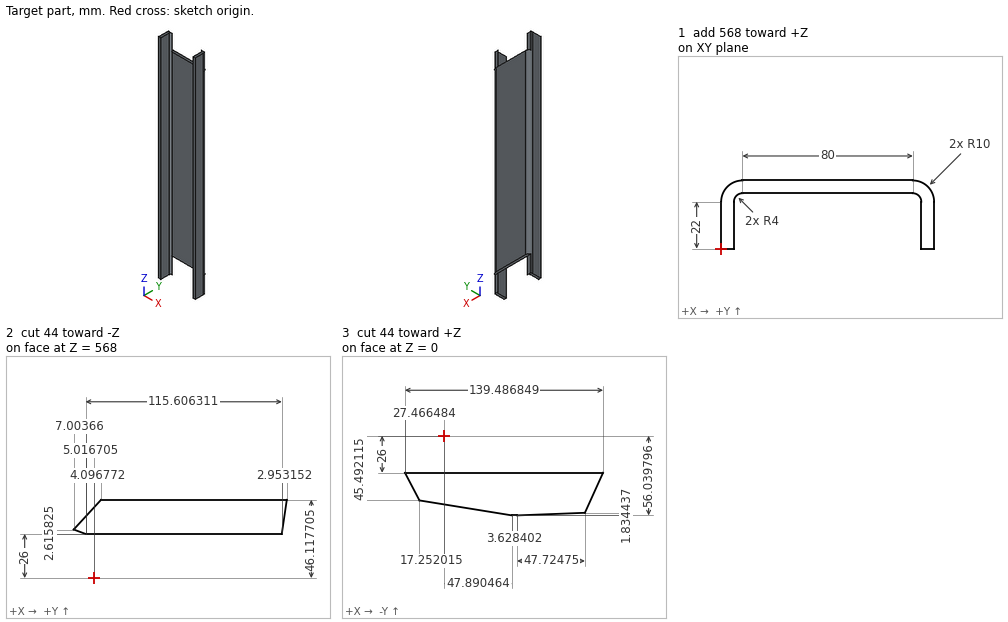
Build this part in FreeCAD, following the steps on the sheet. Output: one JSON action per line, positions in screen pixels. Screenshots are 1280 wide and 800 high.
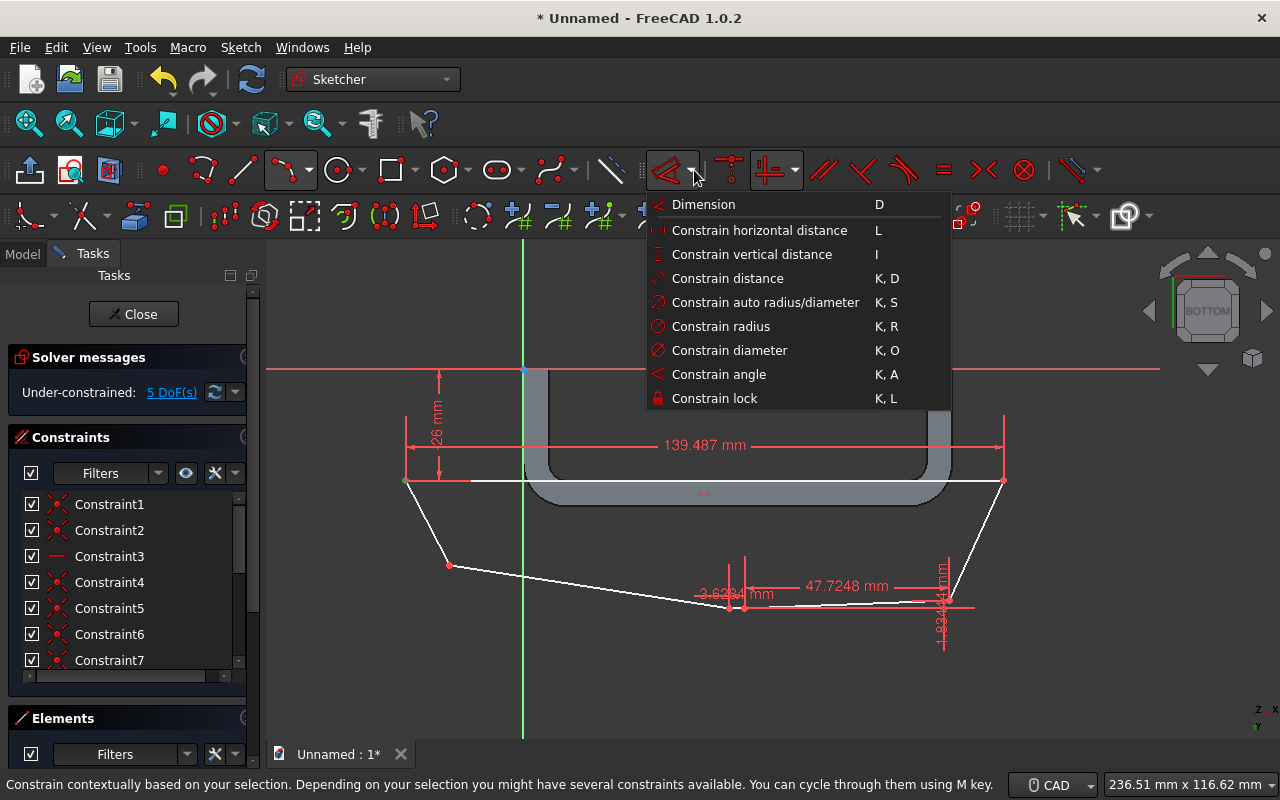
{"action": "left_click", "coordinate": [799, 230]}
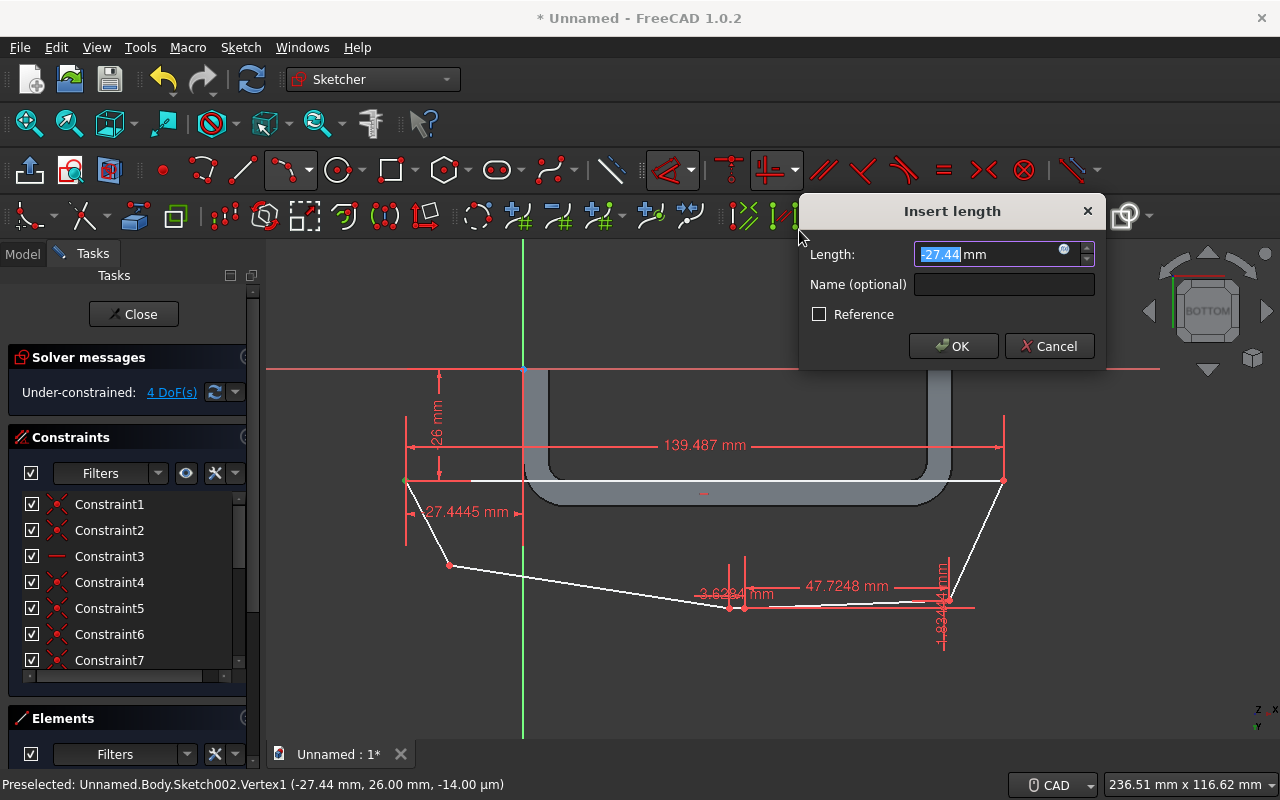
{"action": "type", "text": "-27.466484"}
{"action": "key", "text": "Return"}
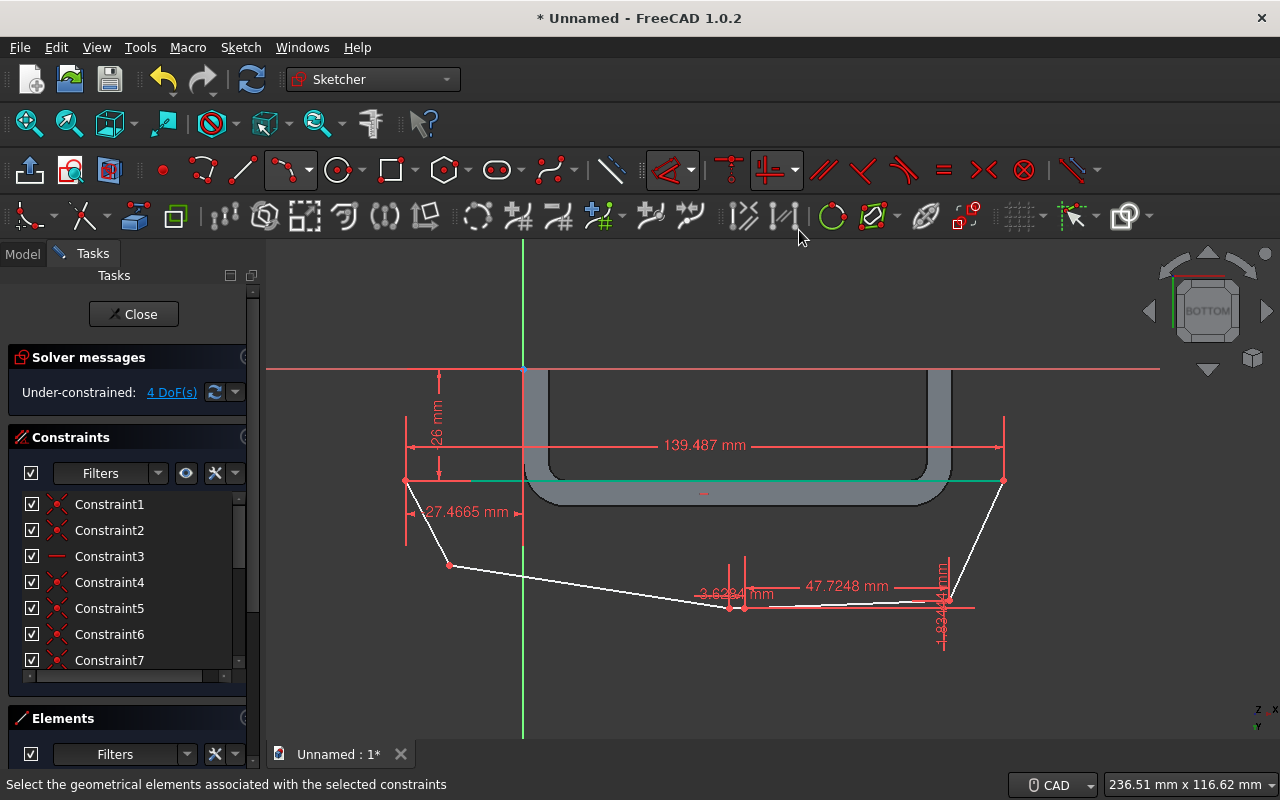
{"action": "left_click", "coordinate": [450, 565]}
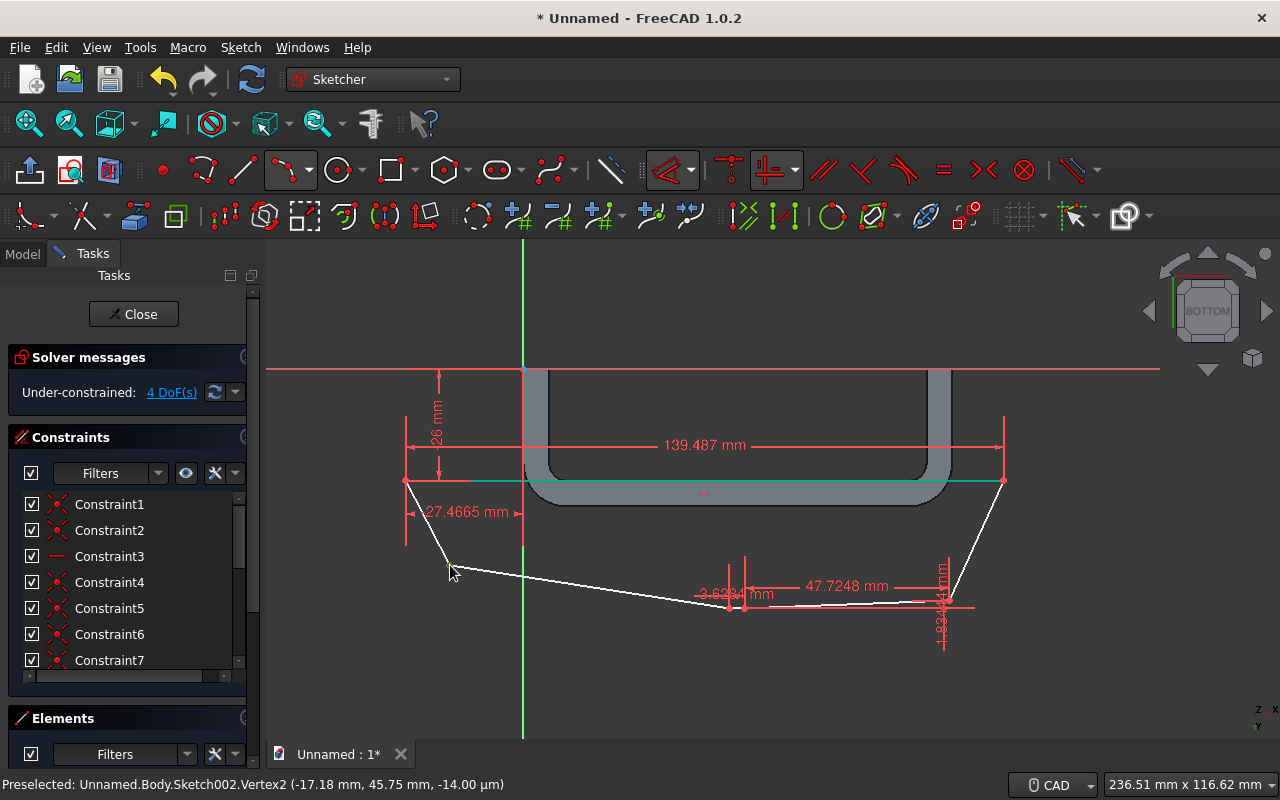
{"action": "key", "text": "l"}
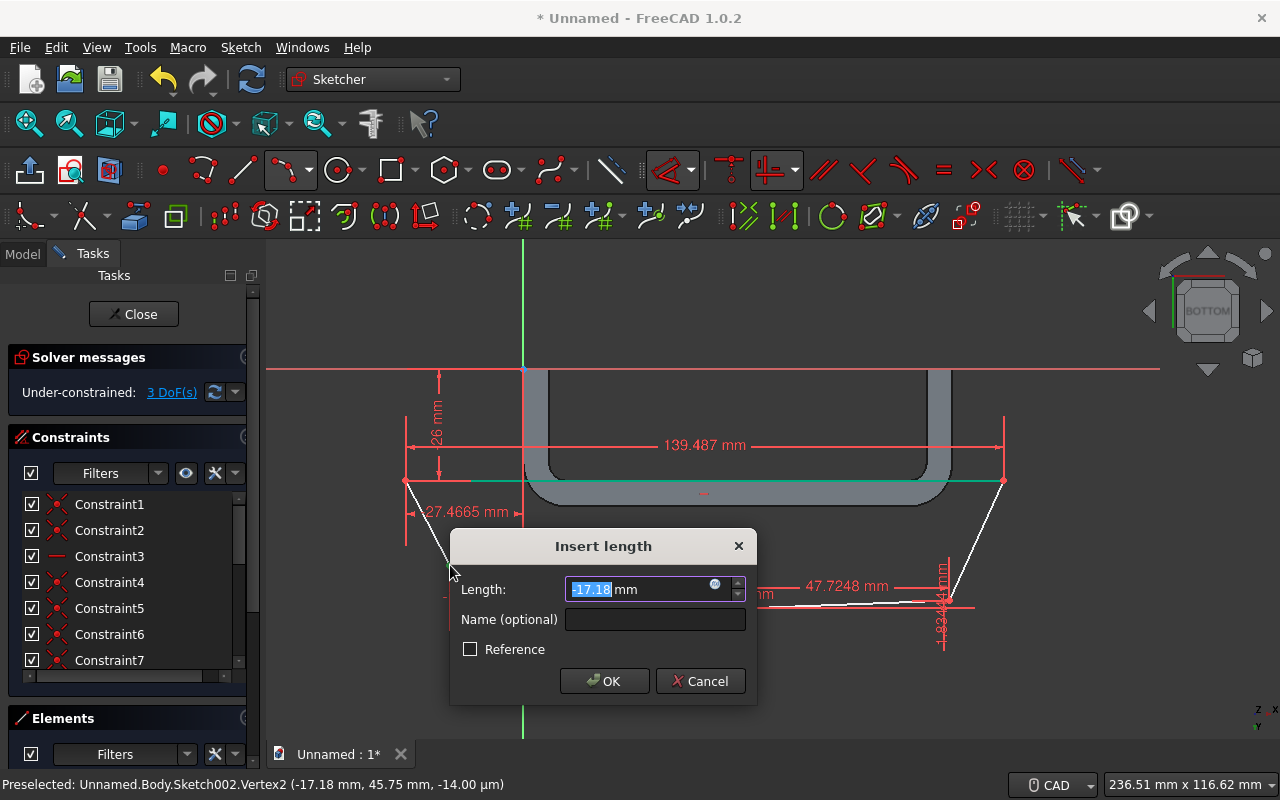
{"action": "type", "text": "-17.252015"}
{"action": "key", "text": "Return"}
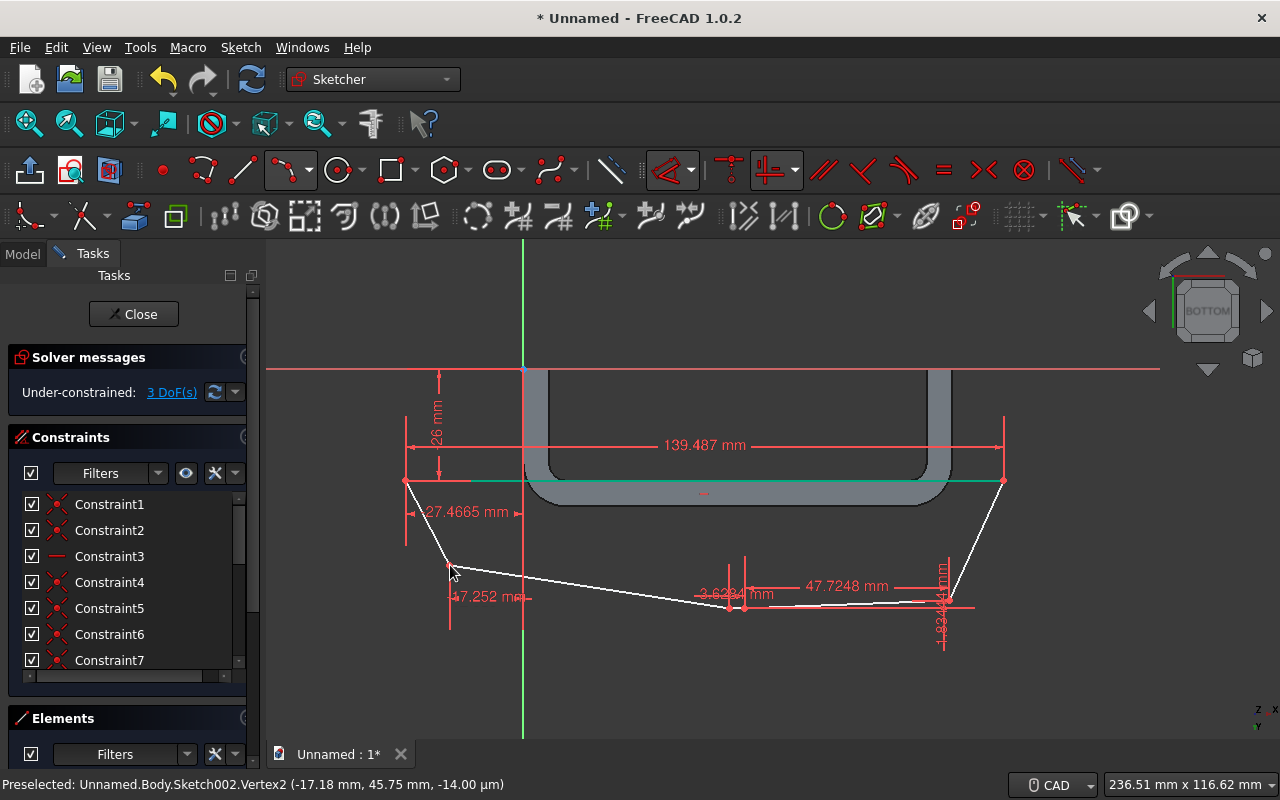
{"action": "left_click", "coordinate": [450, 565]}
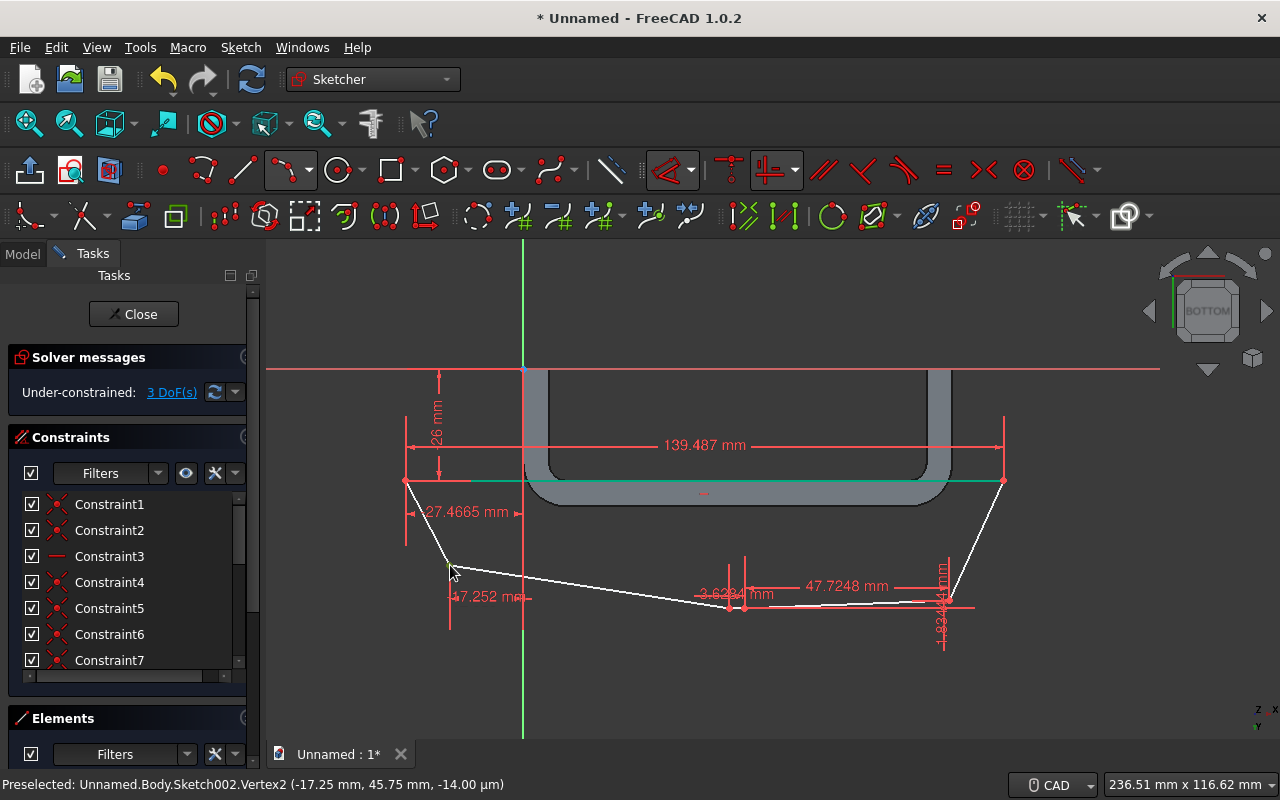
{"action": "key", "text": "i"}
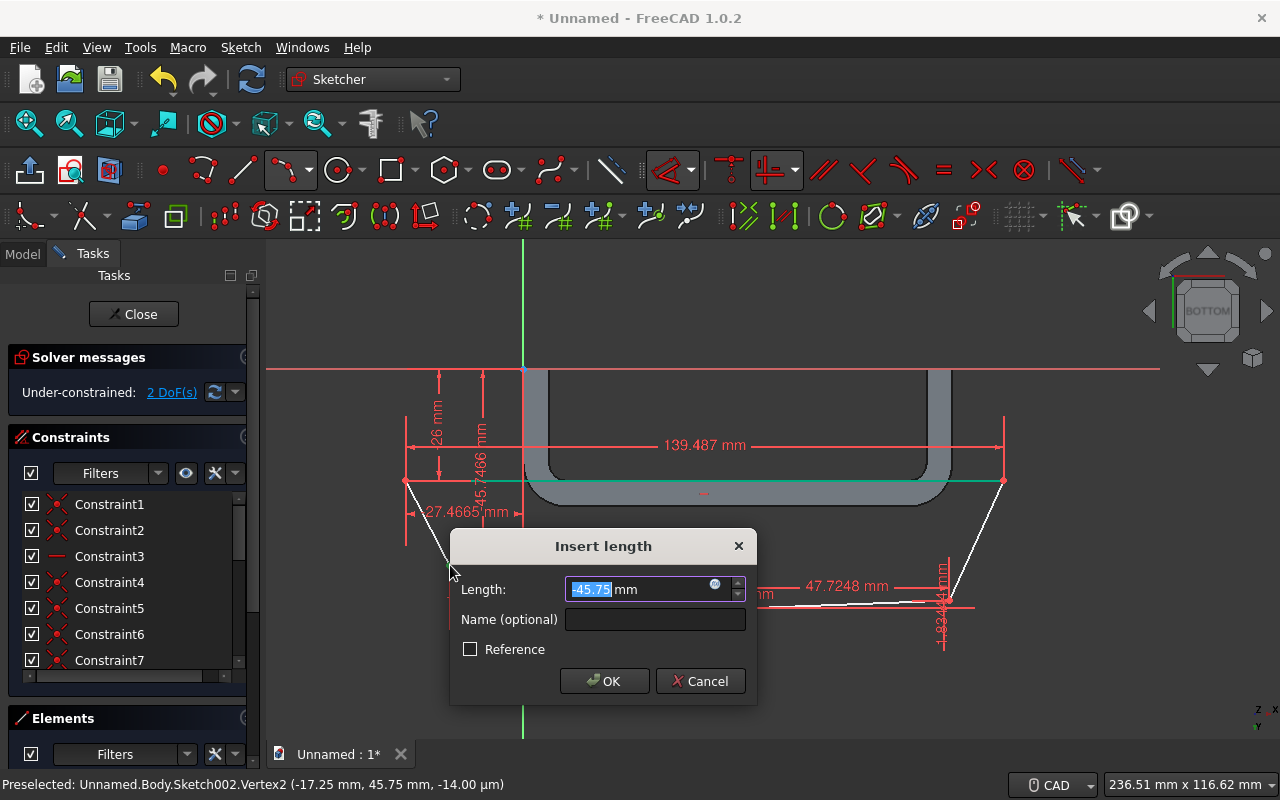
{"action": "type", "text": "-45.492115"}
{"action": "key", "text": "Return"}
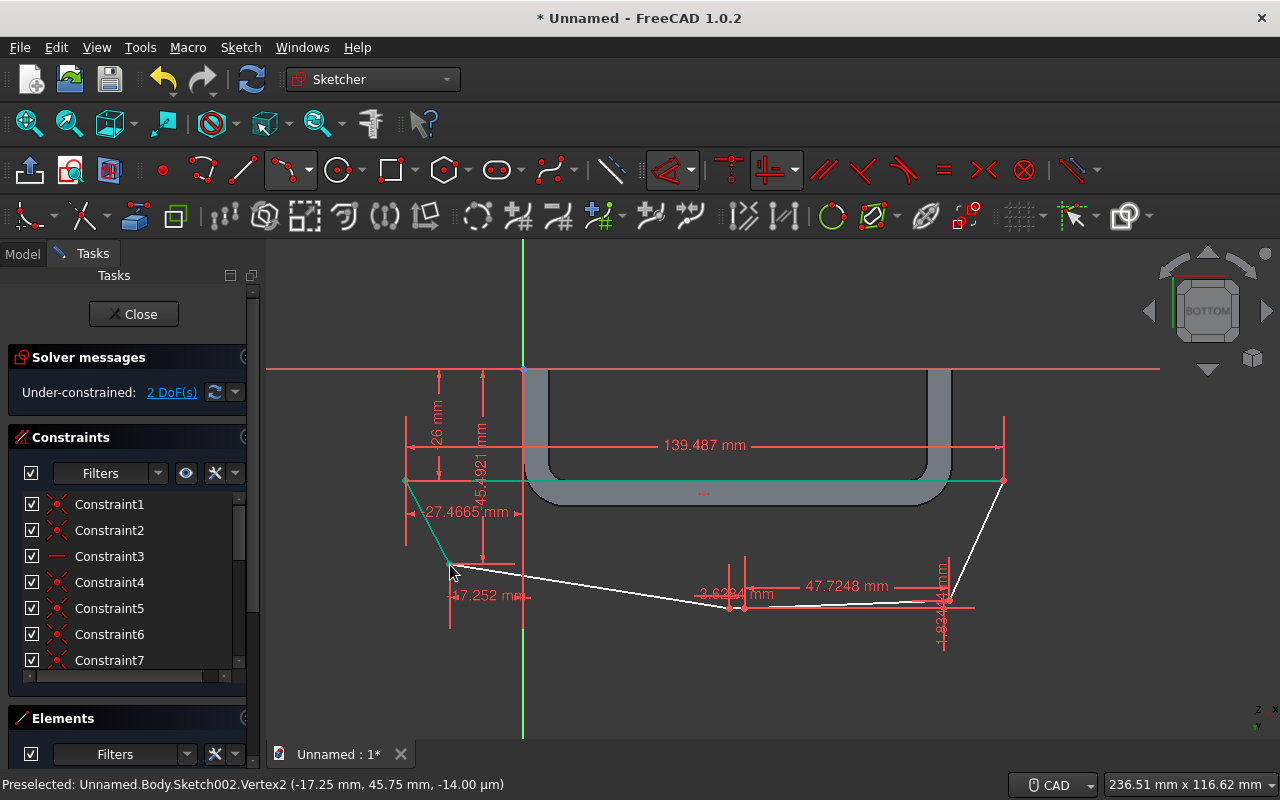
{"action": "left_click", "coordinate": [729, 608]}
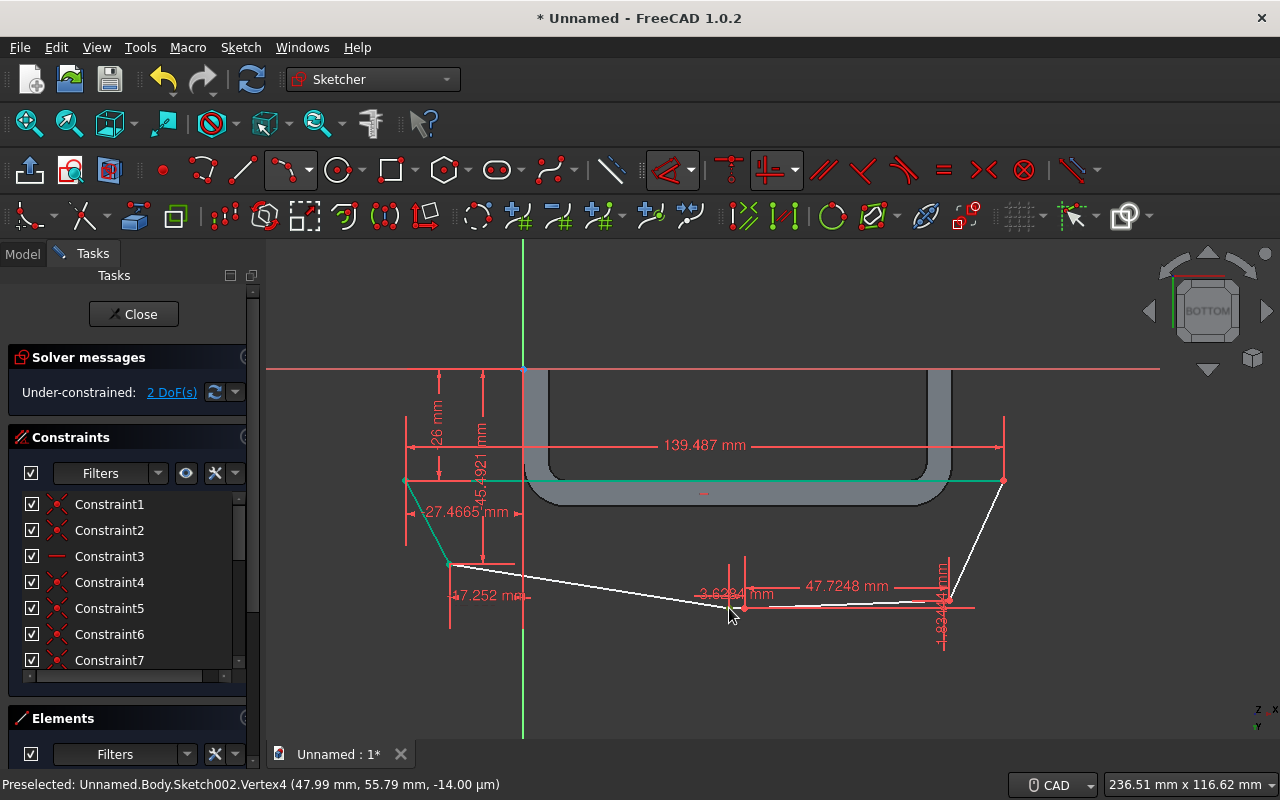
{"action": "key", "text": "l"}